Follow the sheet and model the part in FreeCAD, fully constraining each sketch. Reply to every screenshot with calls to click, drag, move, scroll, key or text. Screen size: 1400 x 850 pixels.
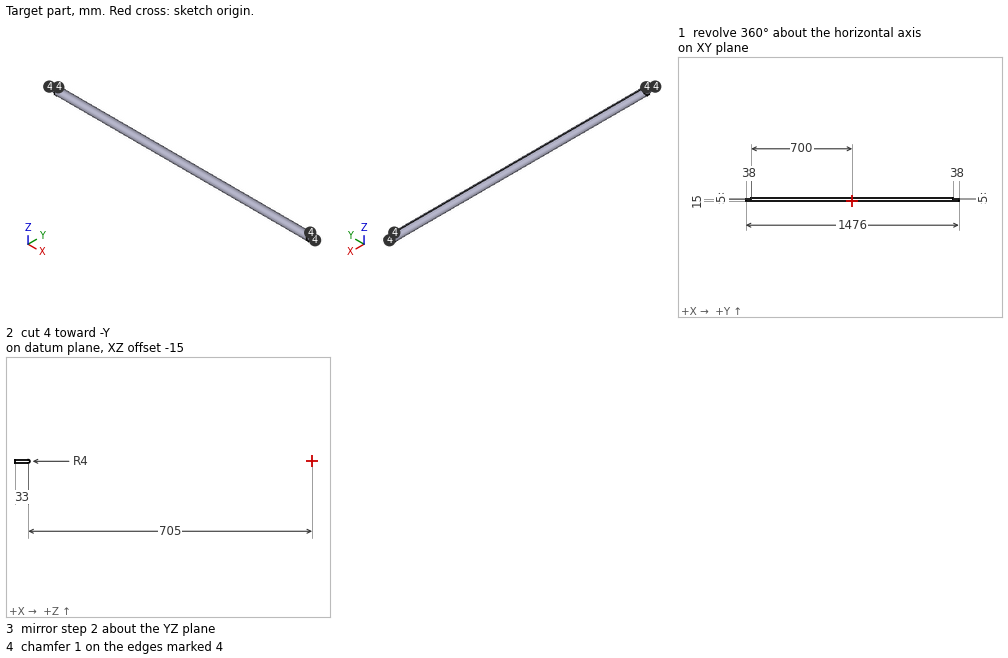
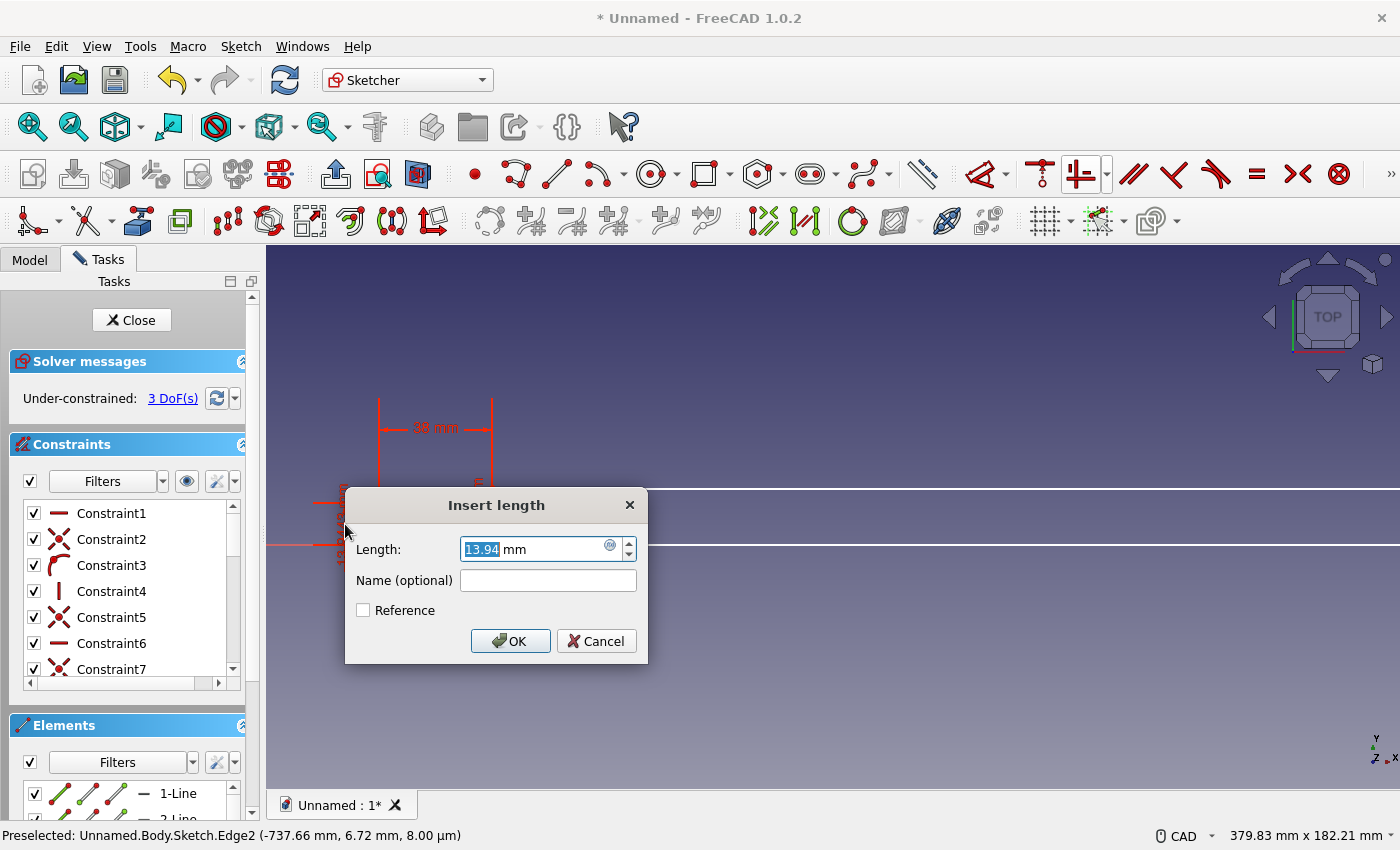
text(15)
key(Return)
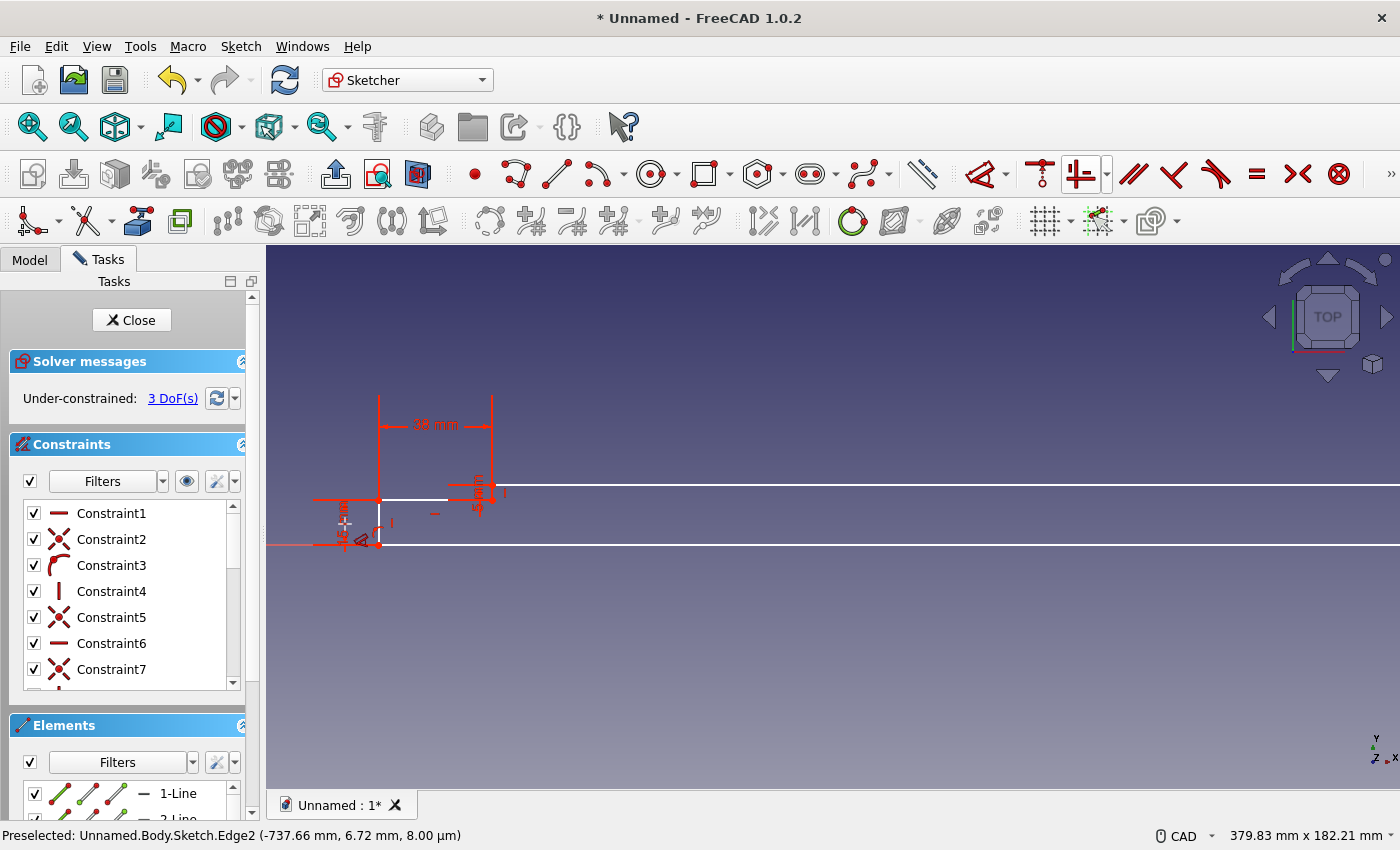
scroll(405, 517, down, 9)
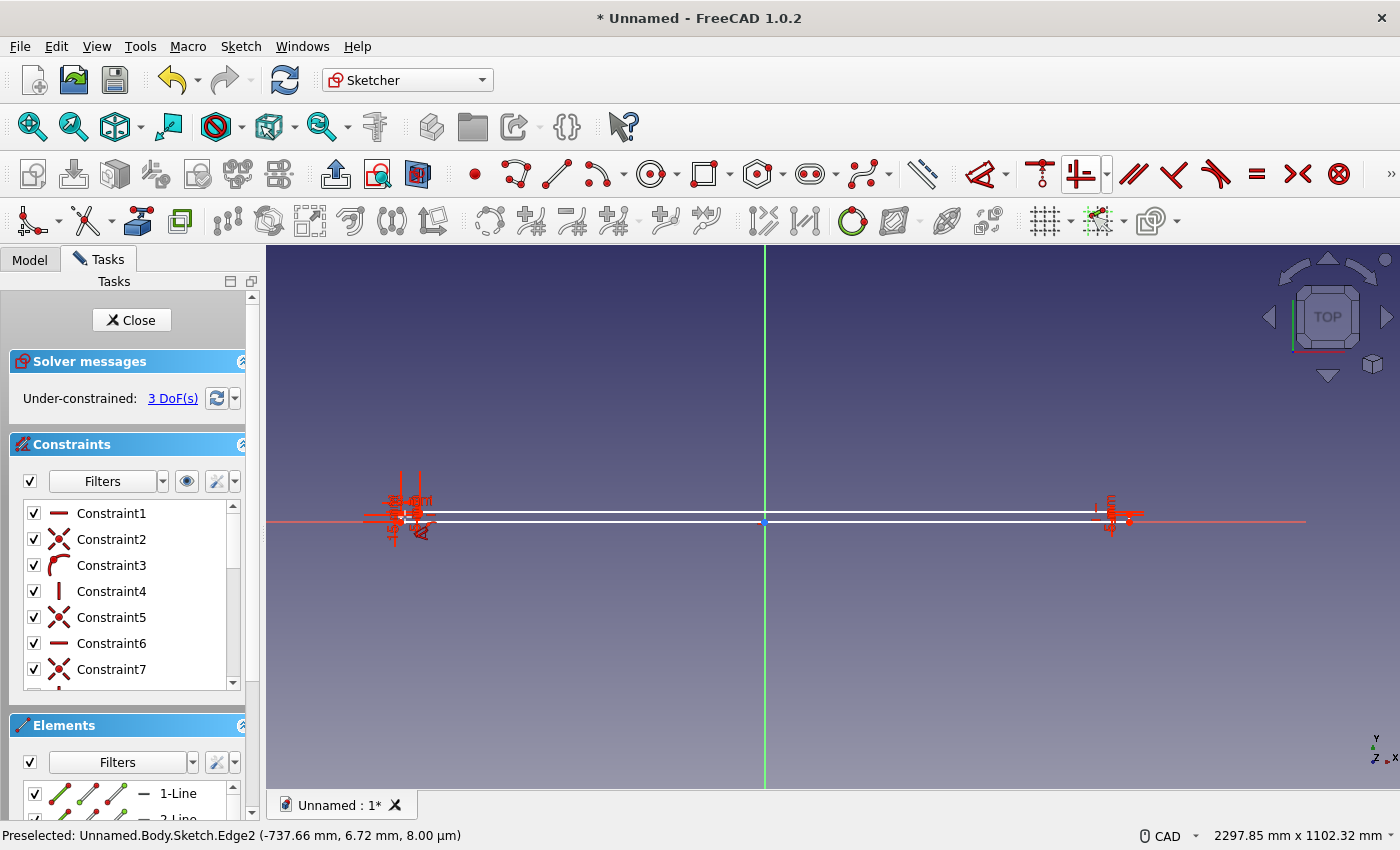
scroll(1123, 515, up, 5)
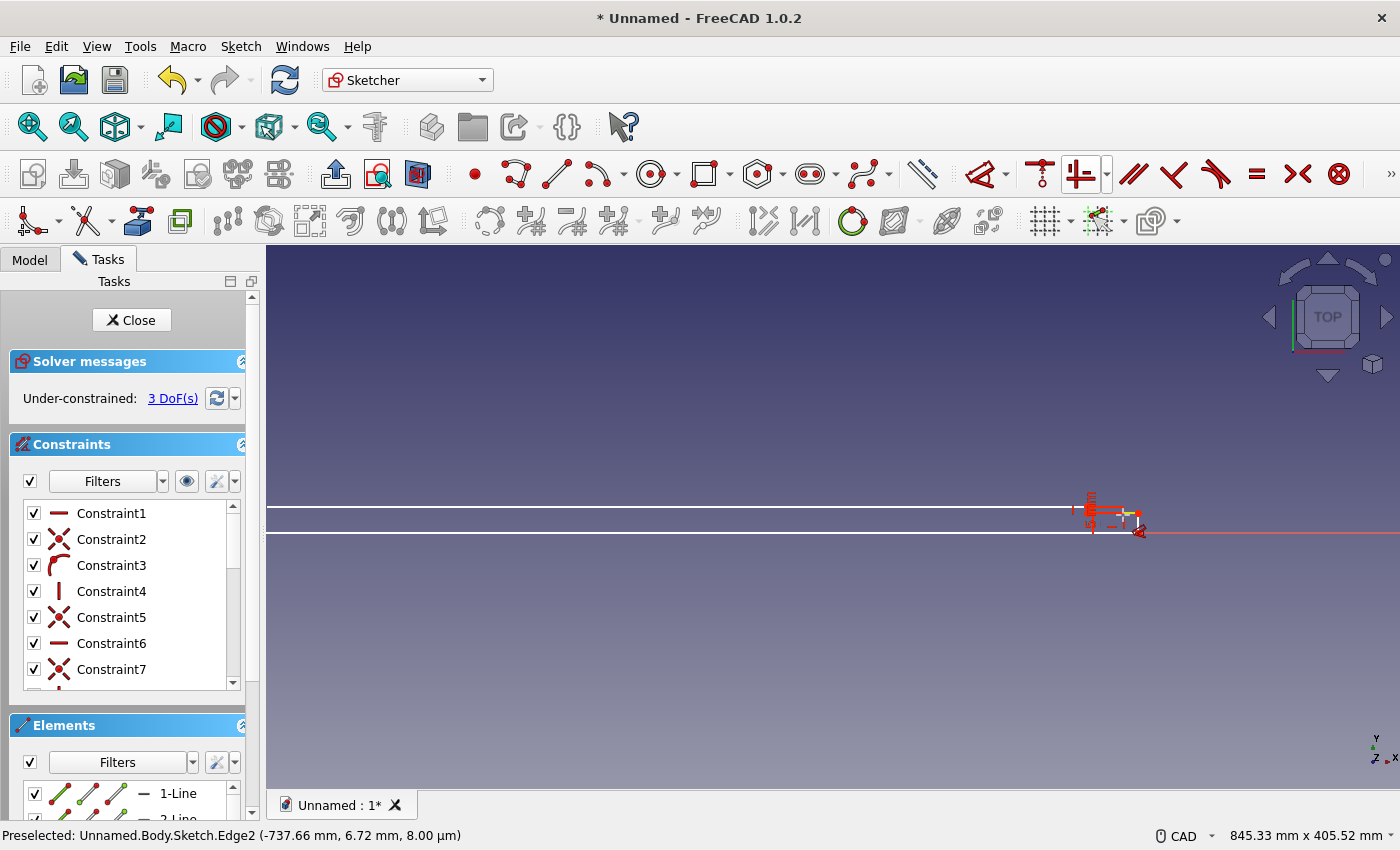
click(1123, 513)
click(1113, 479)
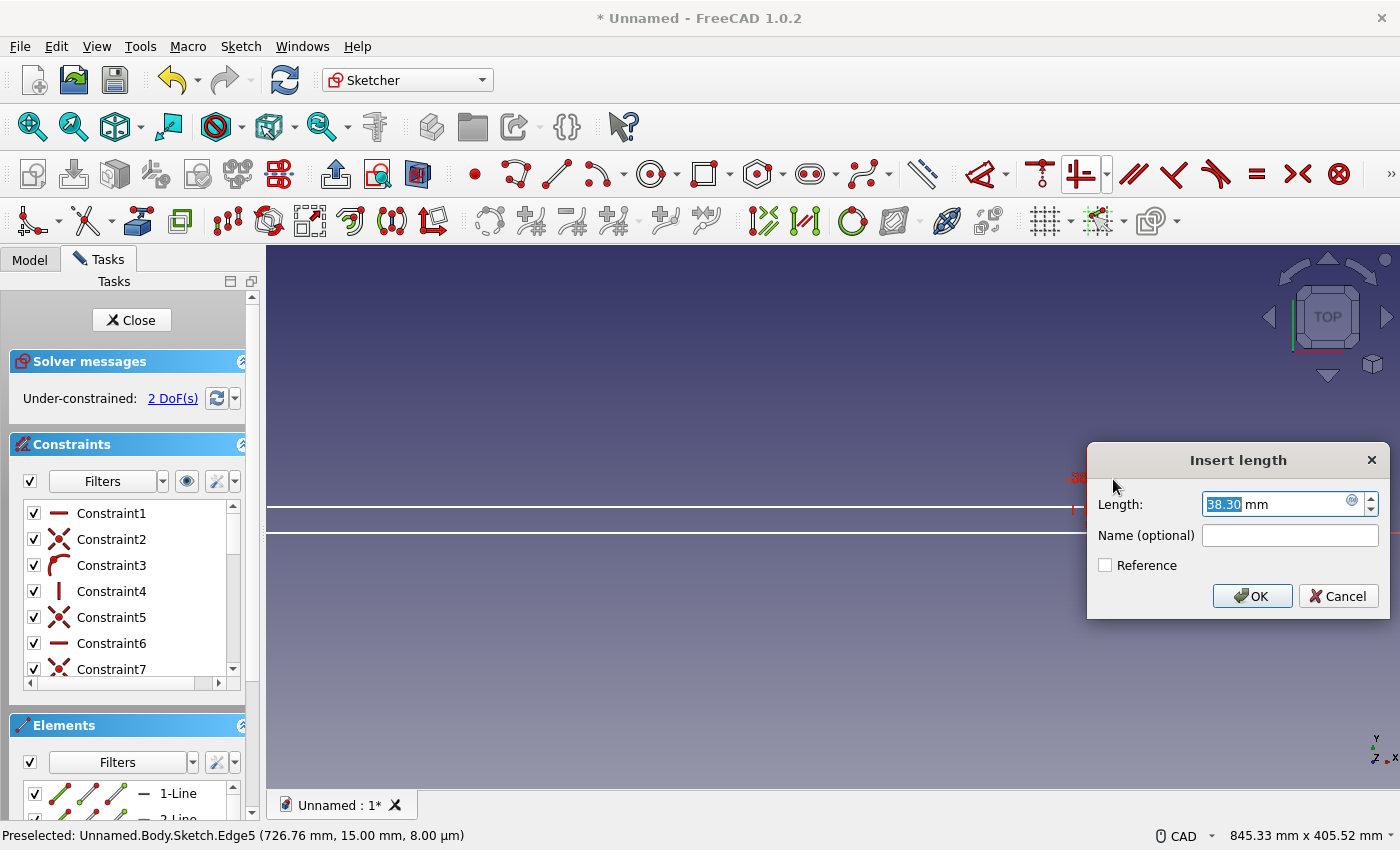
text(38)
key(Return)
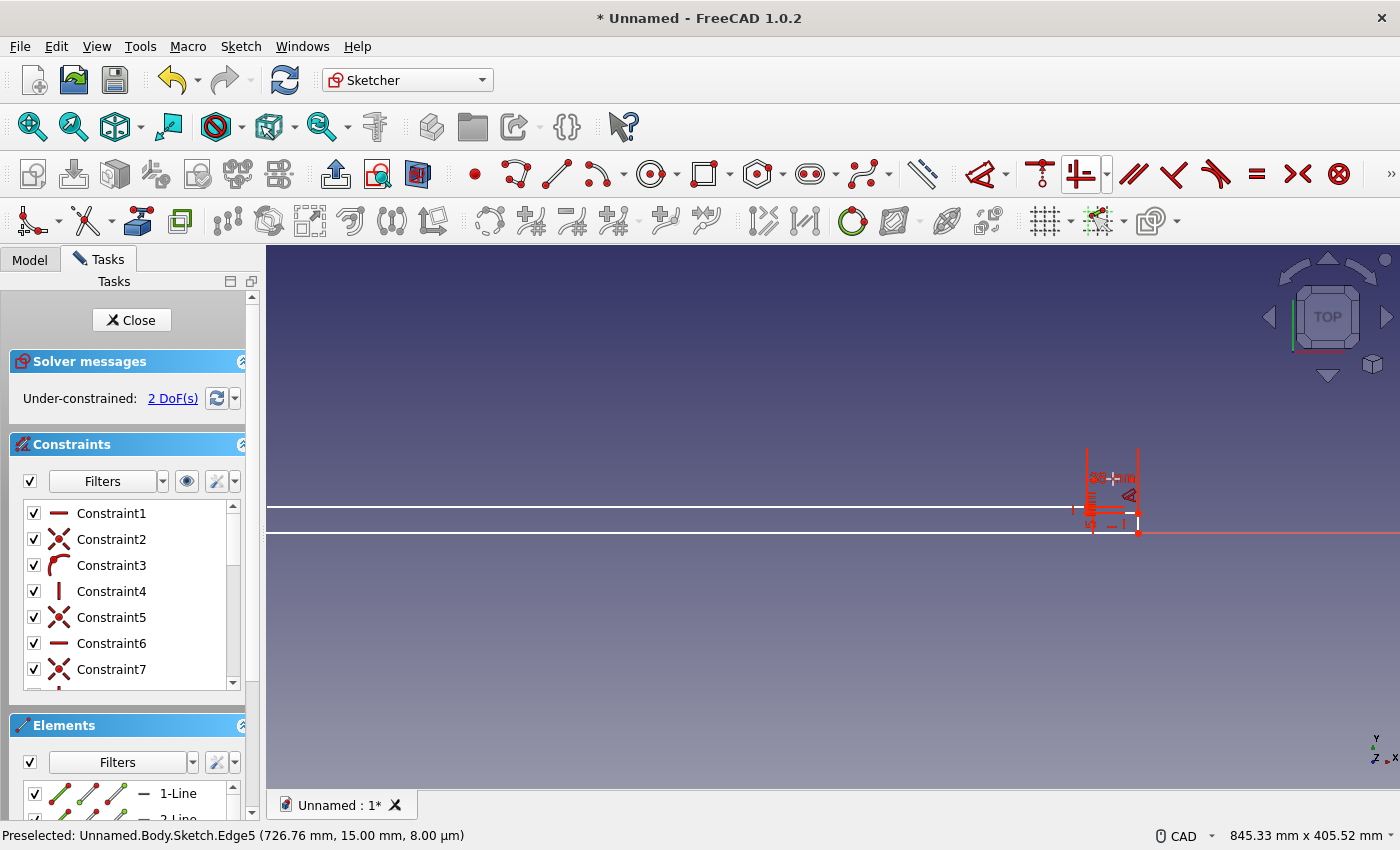
click(544, 533)
click(716, 567)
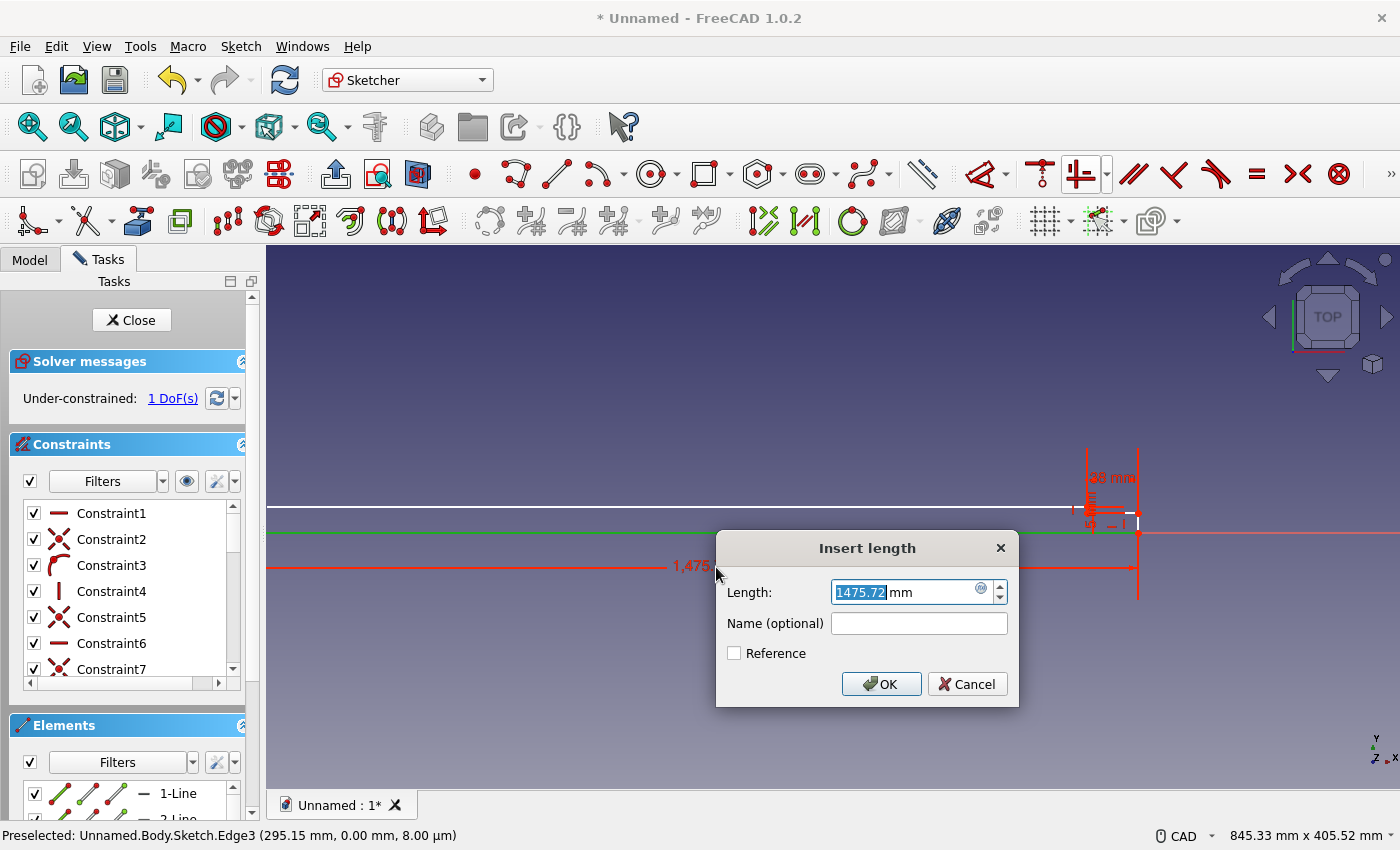
text(1476)
key(Return)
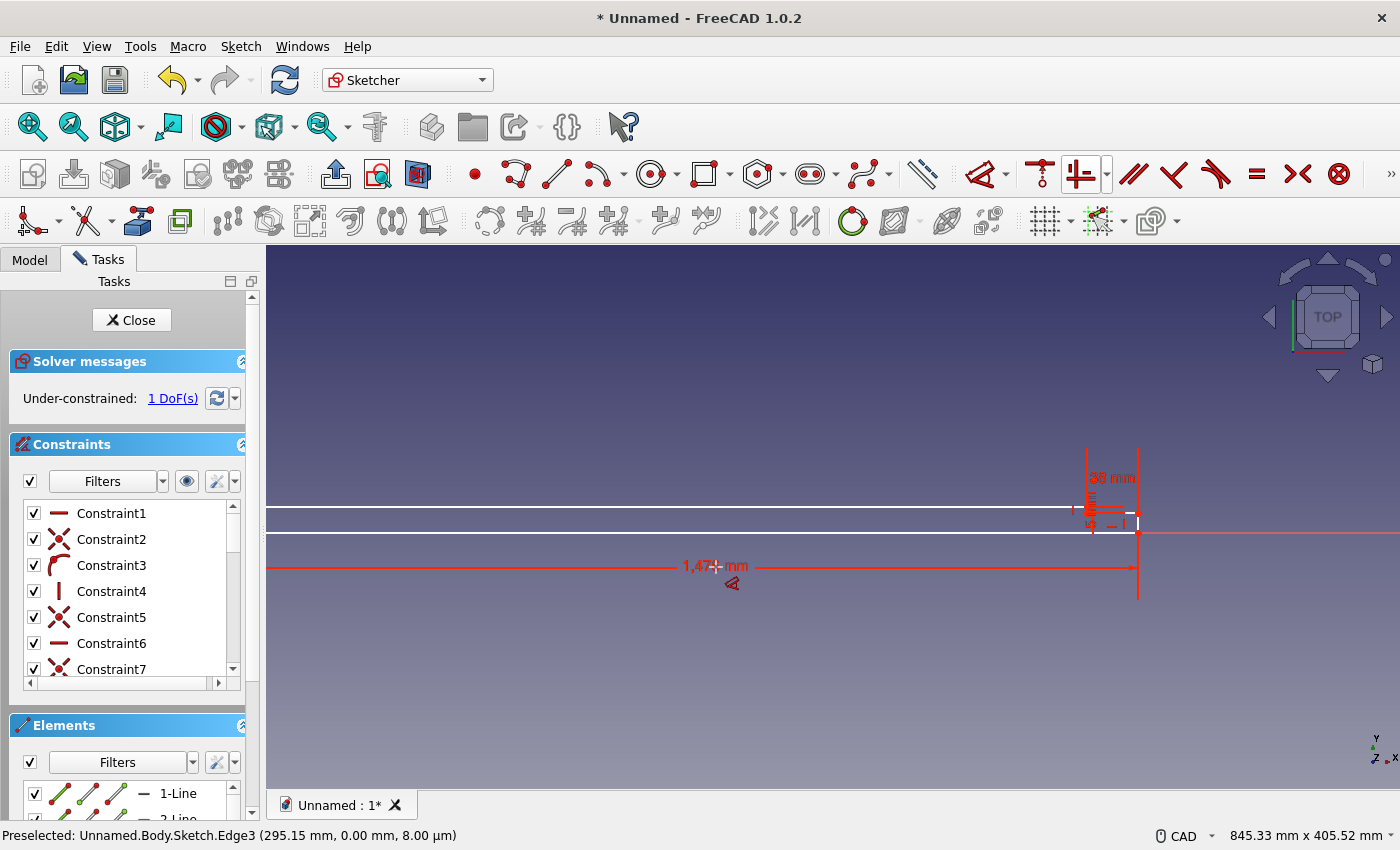
scroll(1123, 515, down, 5)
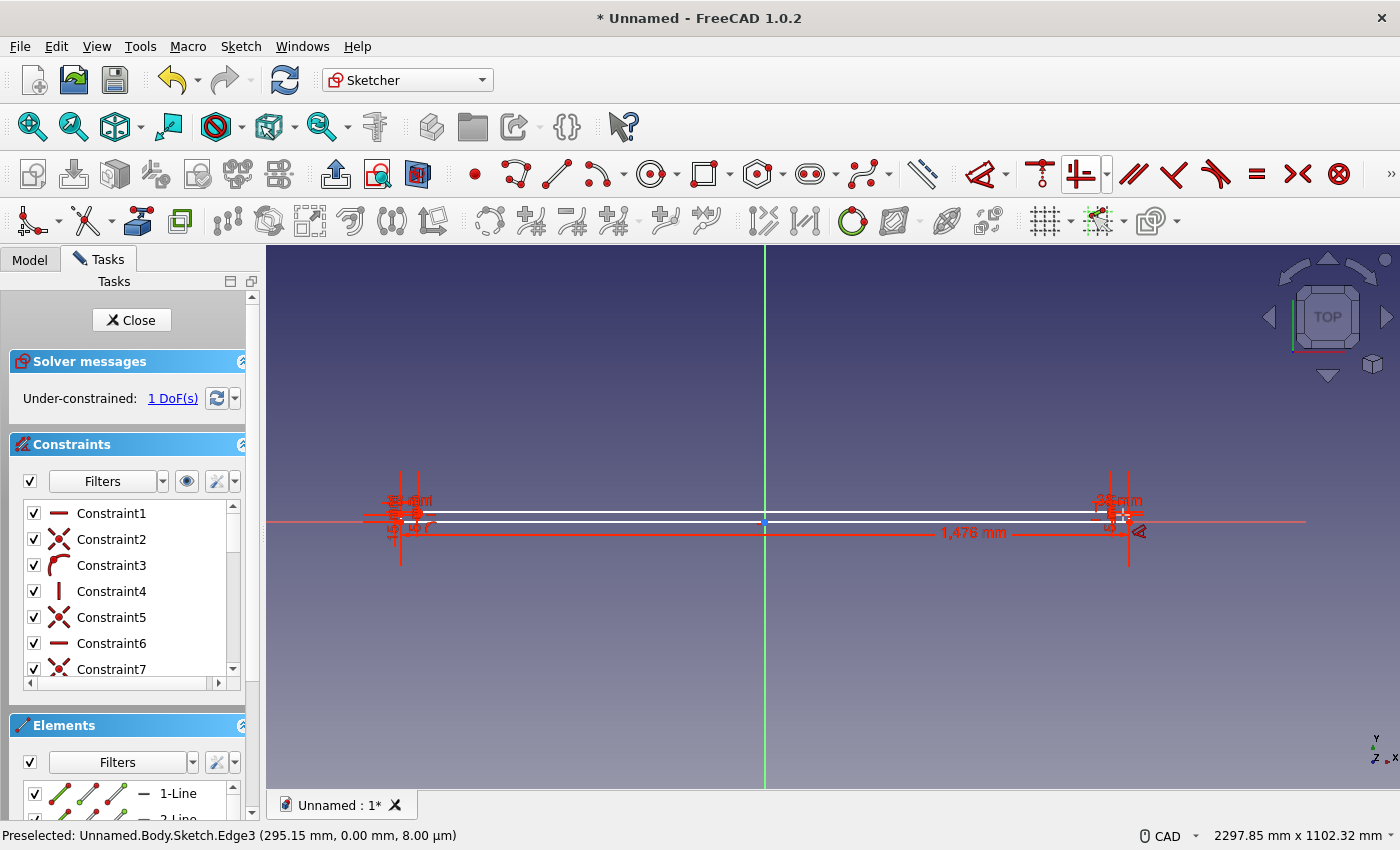
scroll(419, 515, up, 8)